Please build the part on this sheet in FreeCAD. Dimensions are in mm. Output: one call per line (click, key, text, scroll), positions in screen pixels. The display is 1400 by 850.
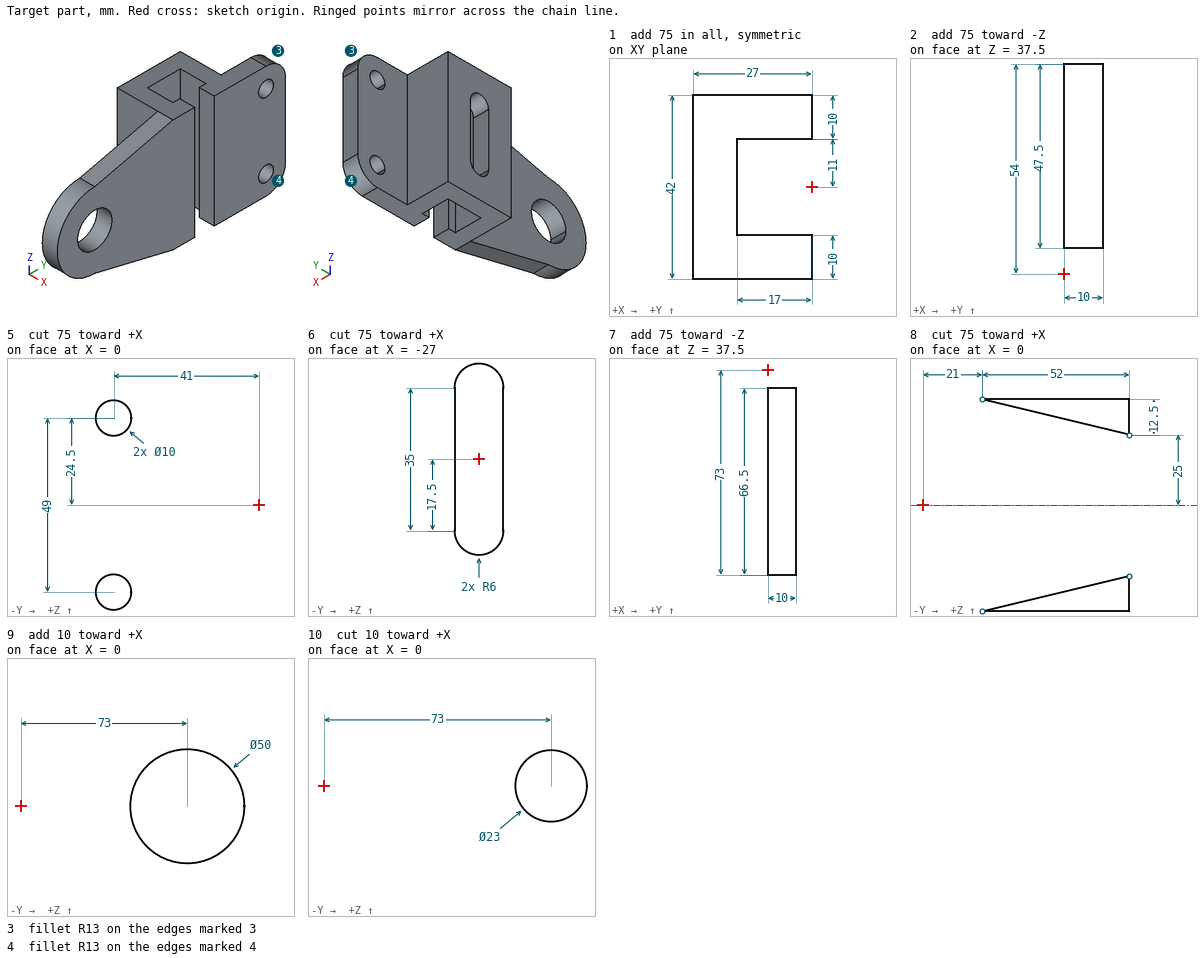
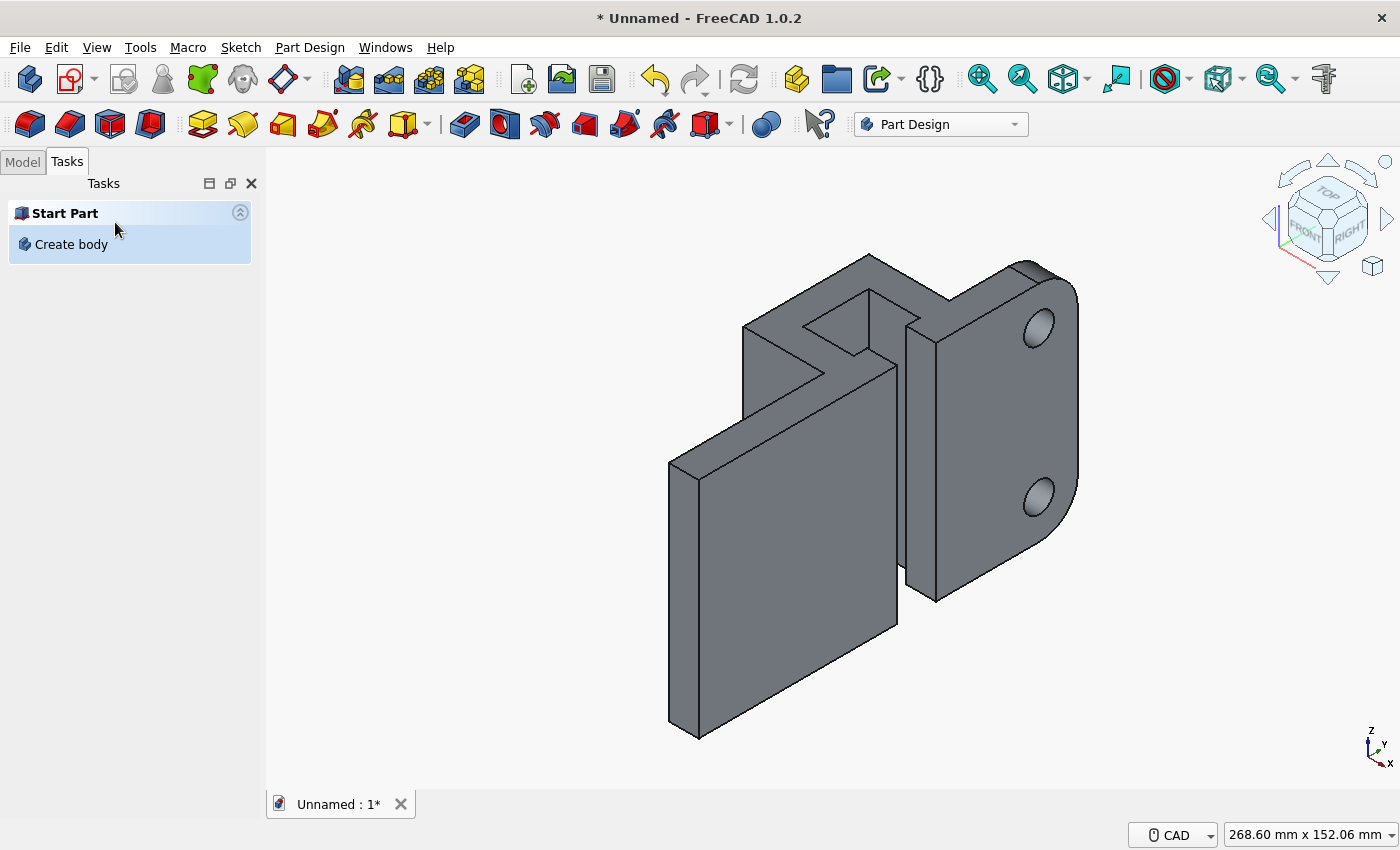
key(6)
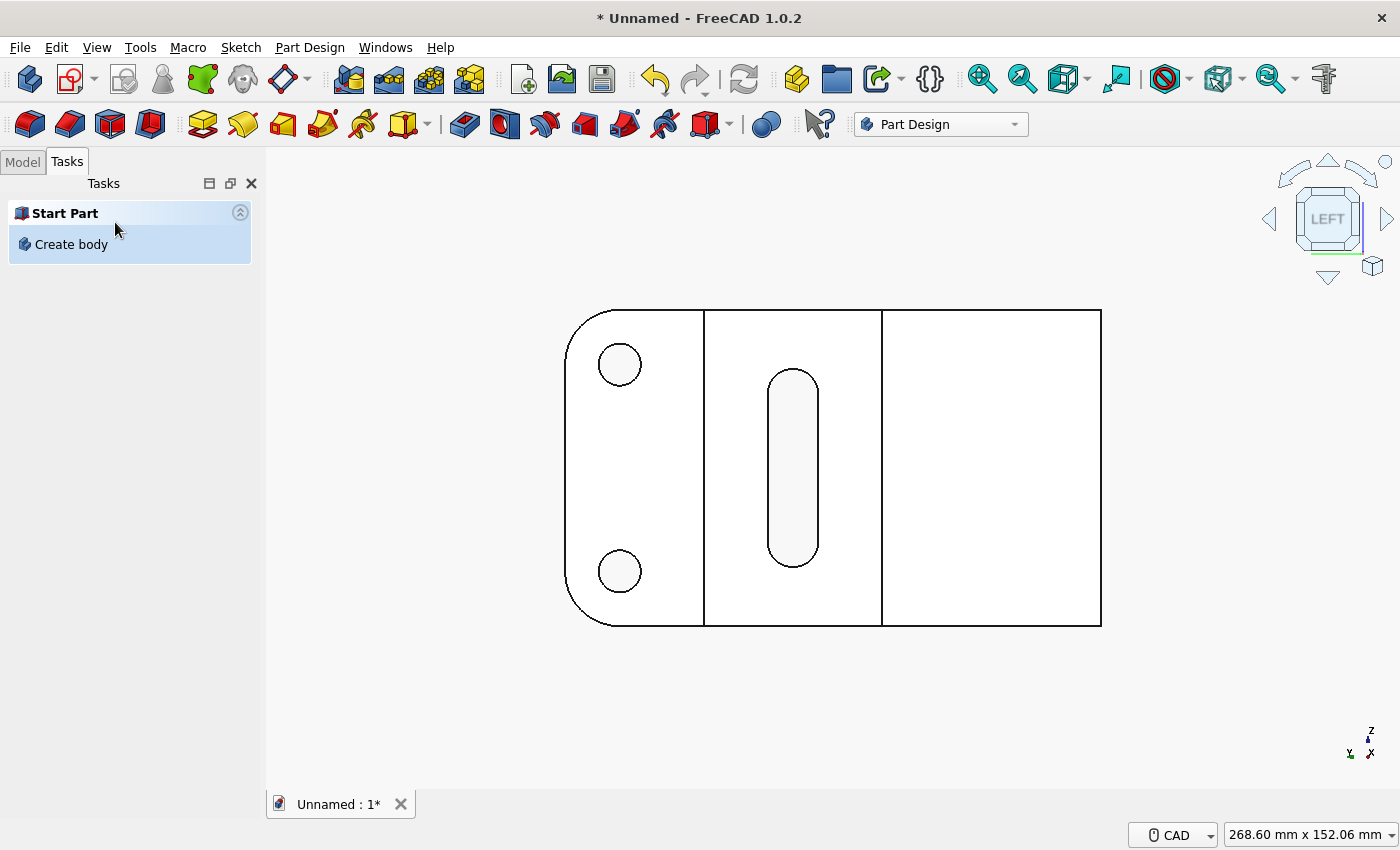
click(991, 422)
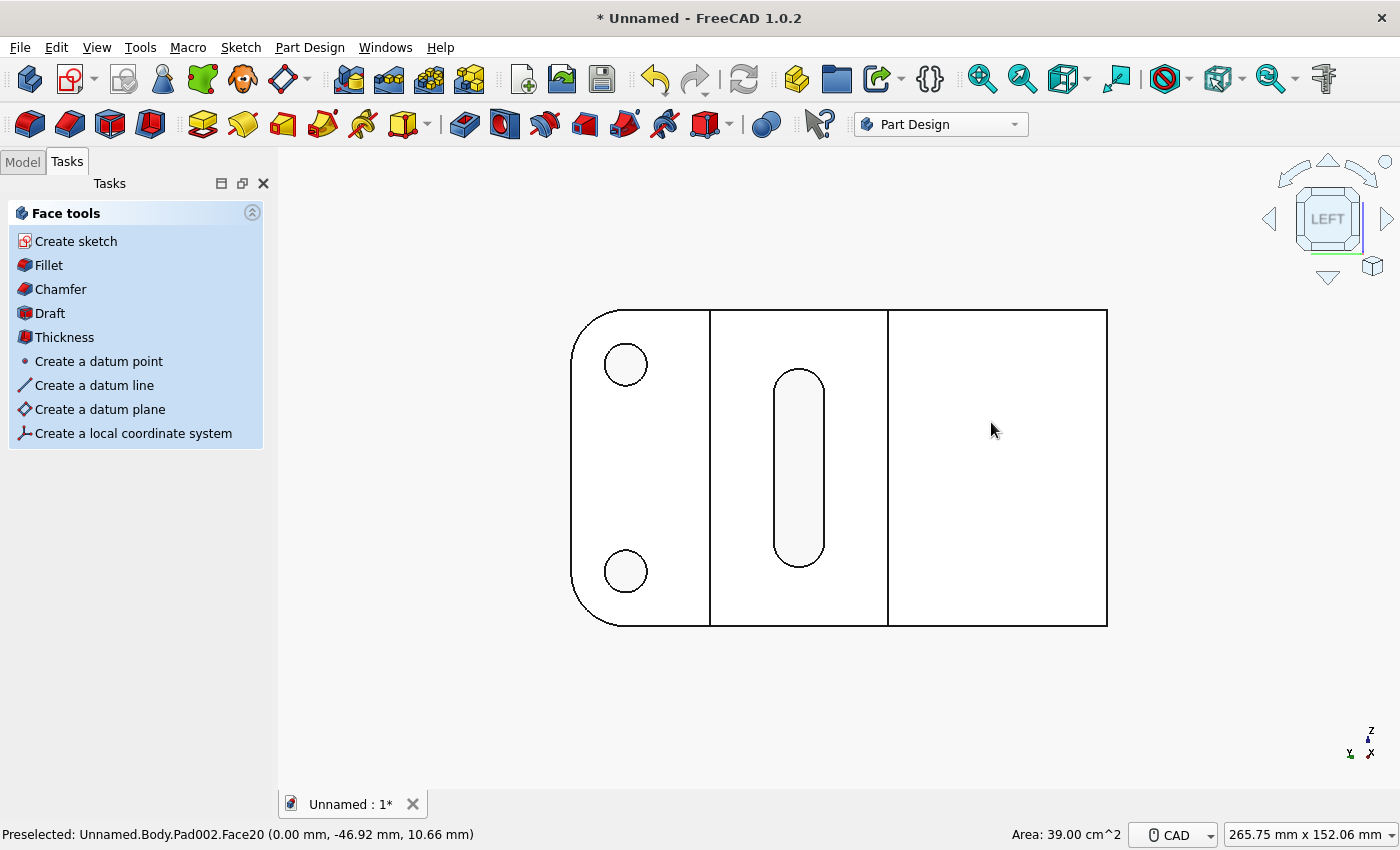
click(70, 80)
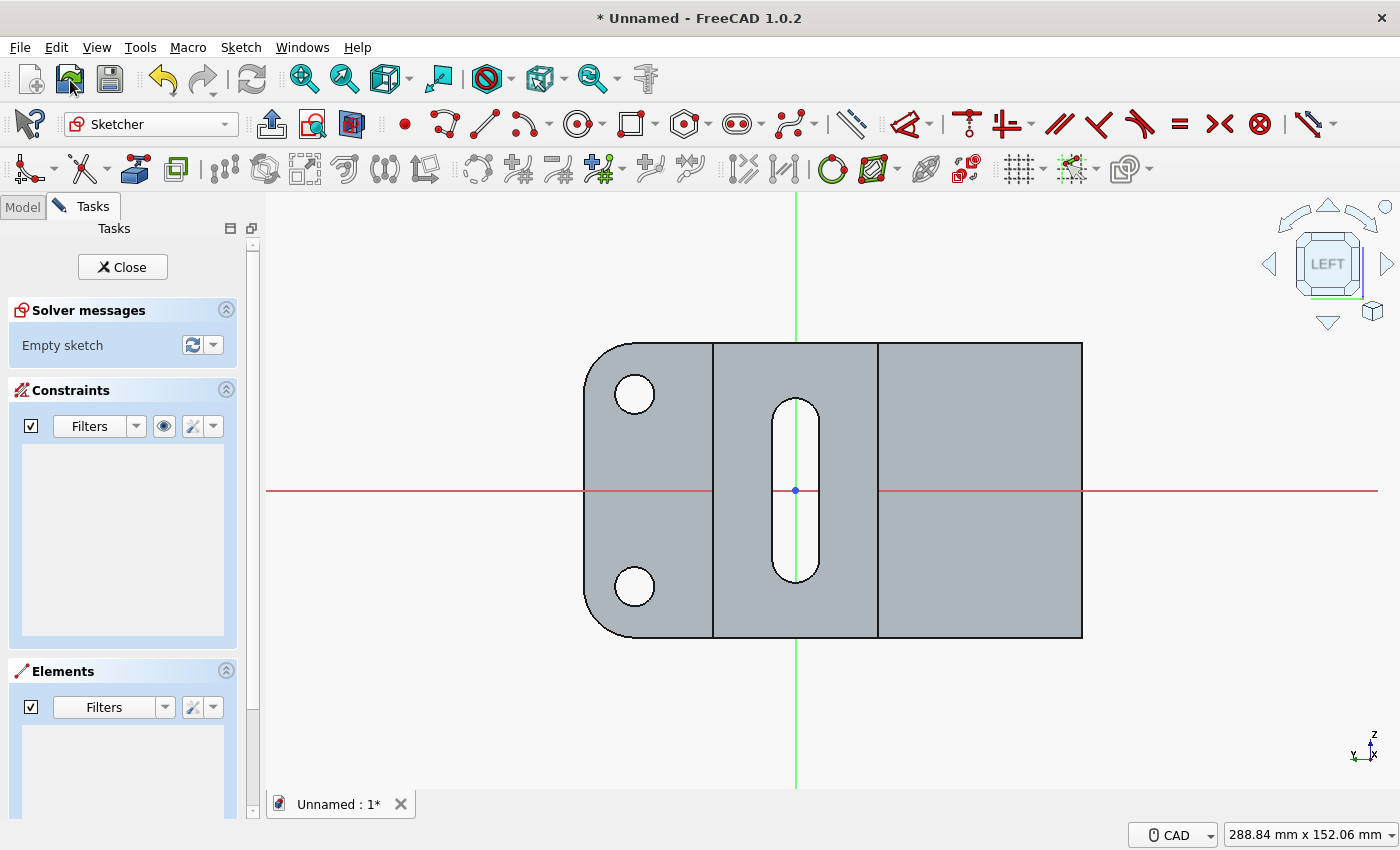
key(q)
key(s)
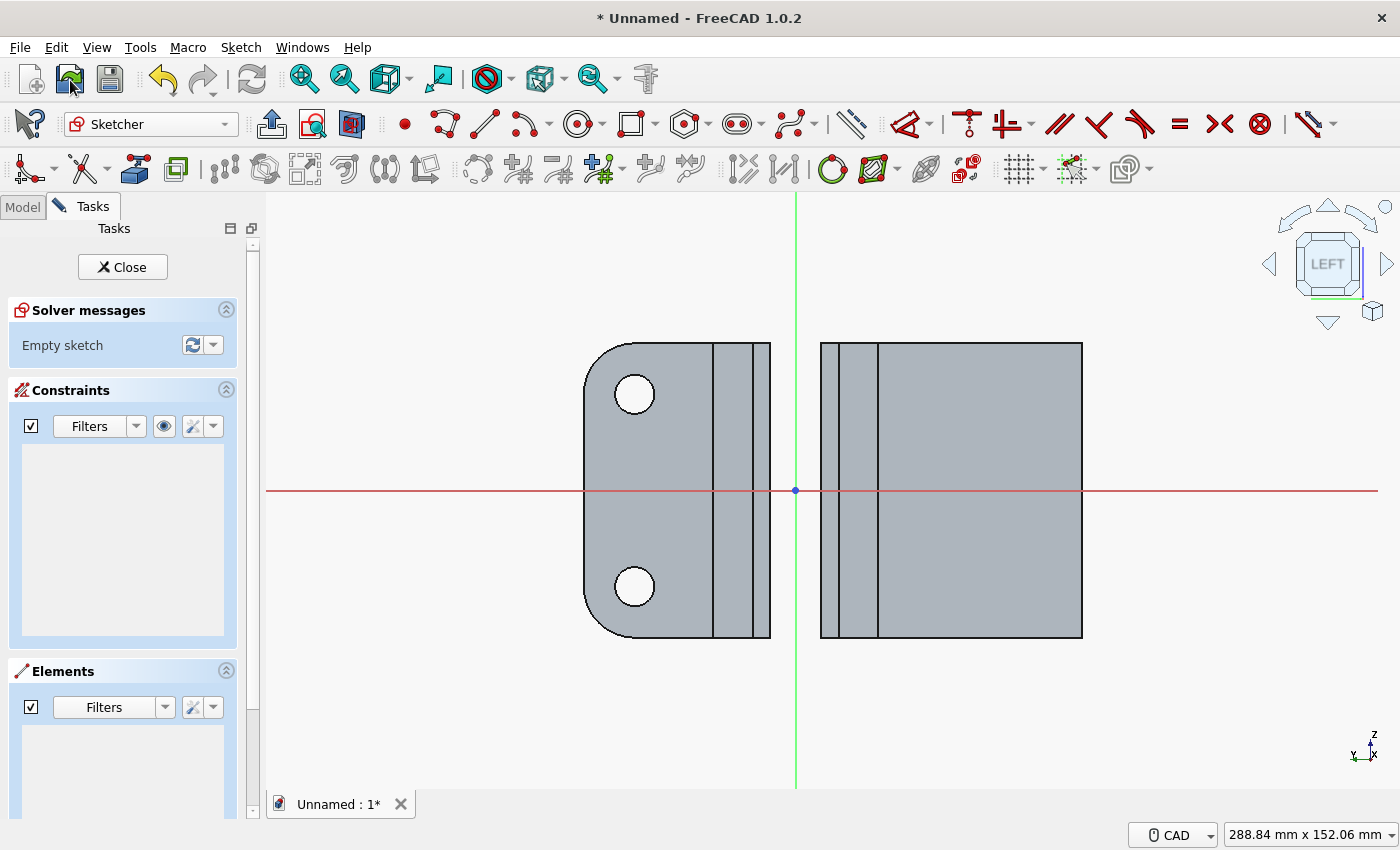
key(g)
key(m)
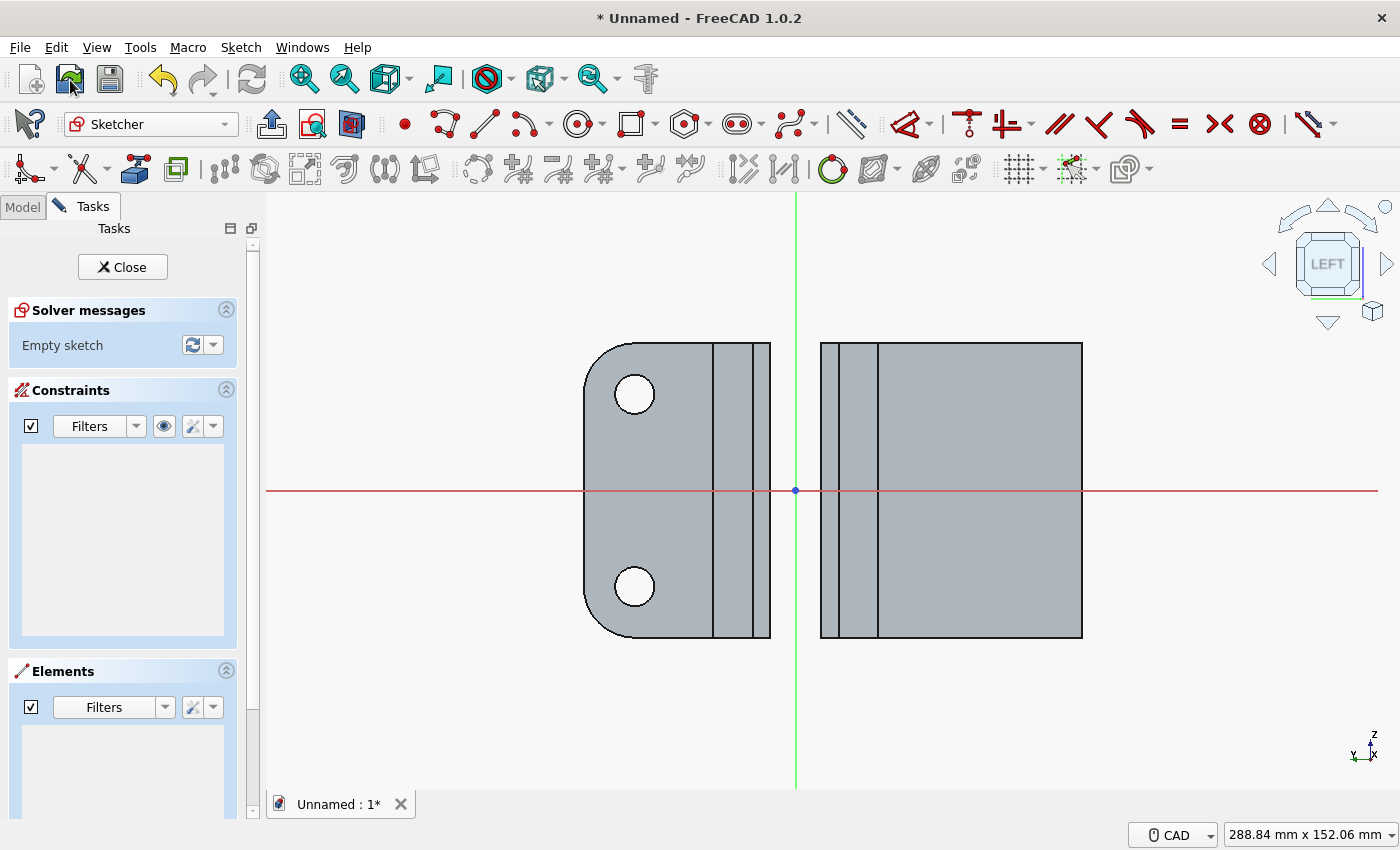
click(878, 343)
click(1082, 392)
click(1082, 343)
click(878, 344)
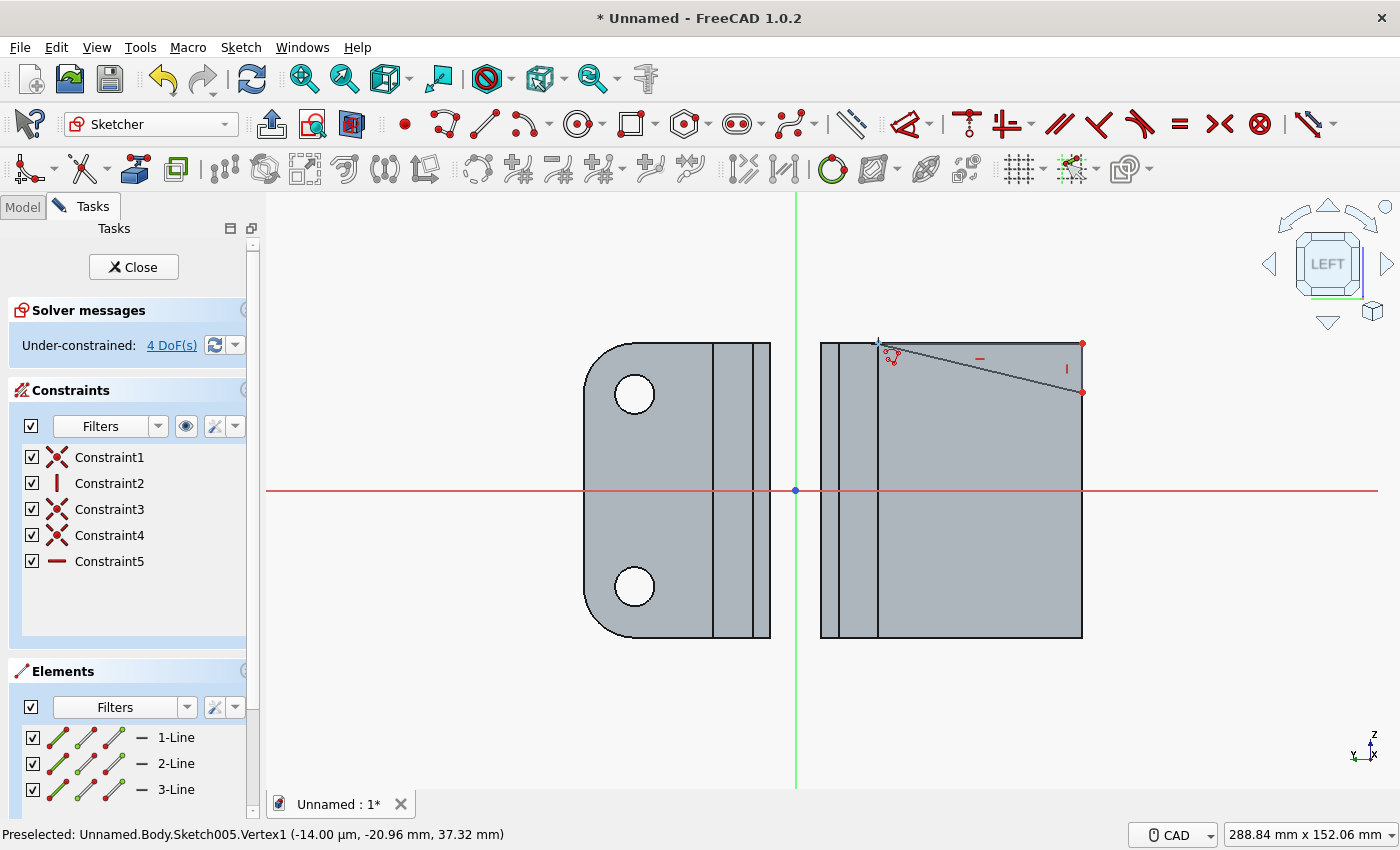
click(878, 638)
click(1082, 638)
click(1082, 589)
click(878, 639)
key(Escape)
key(Escape)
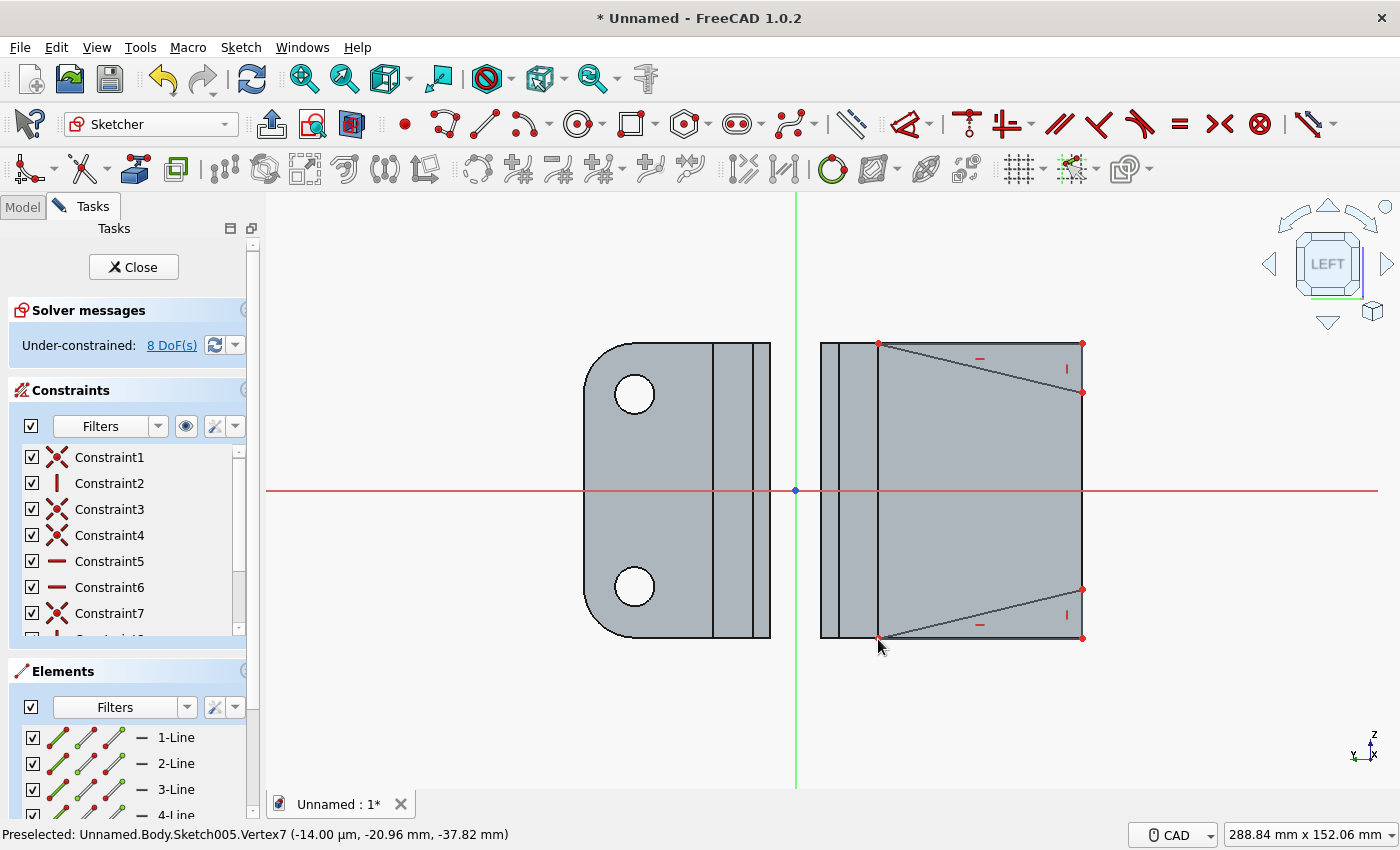
click(878, 344)